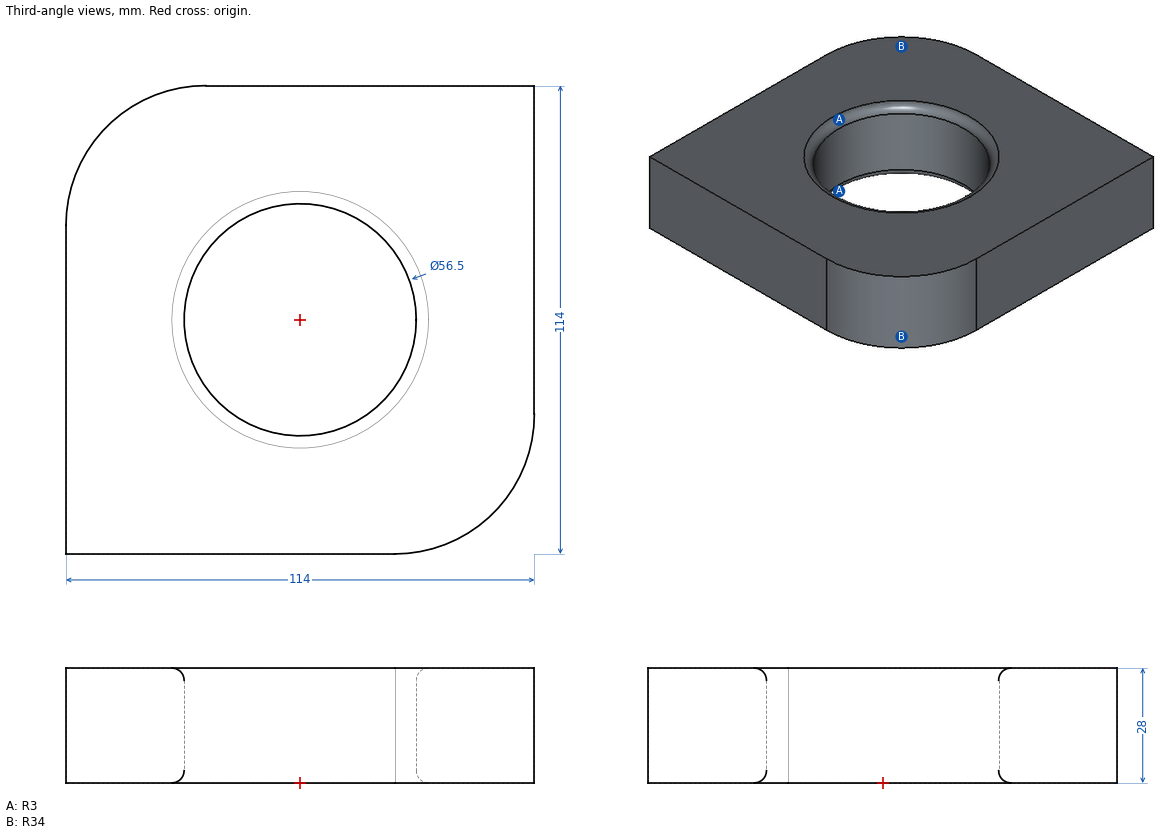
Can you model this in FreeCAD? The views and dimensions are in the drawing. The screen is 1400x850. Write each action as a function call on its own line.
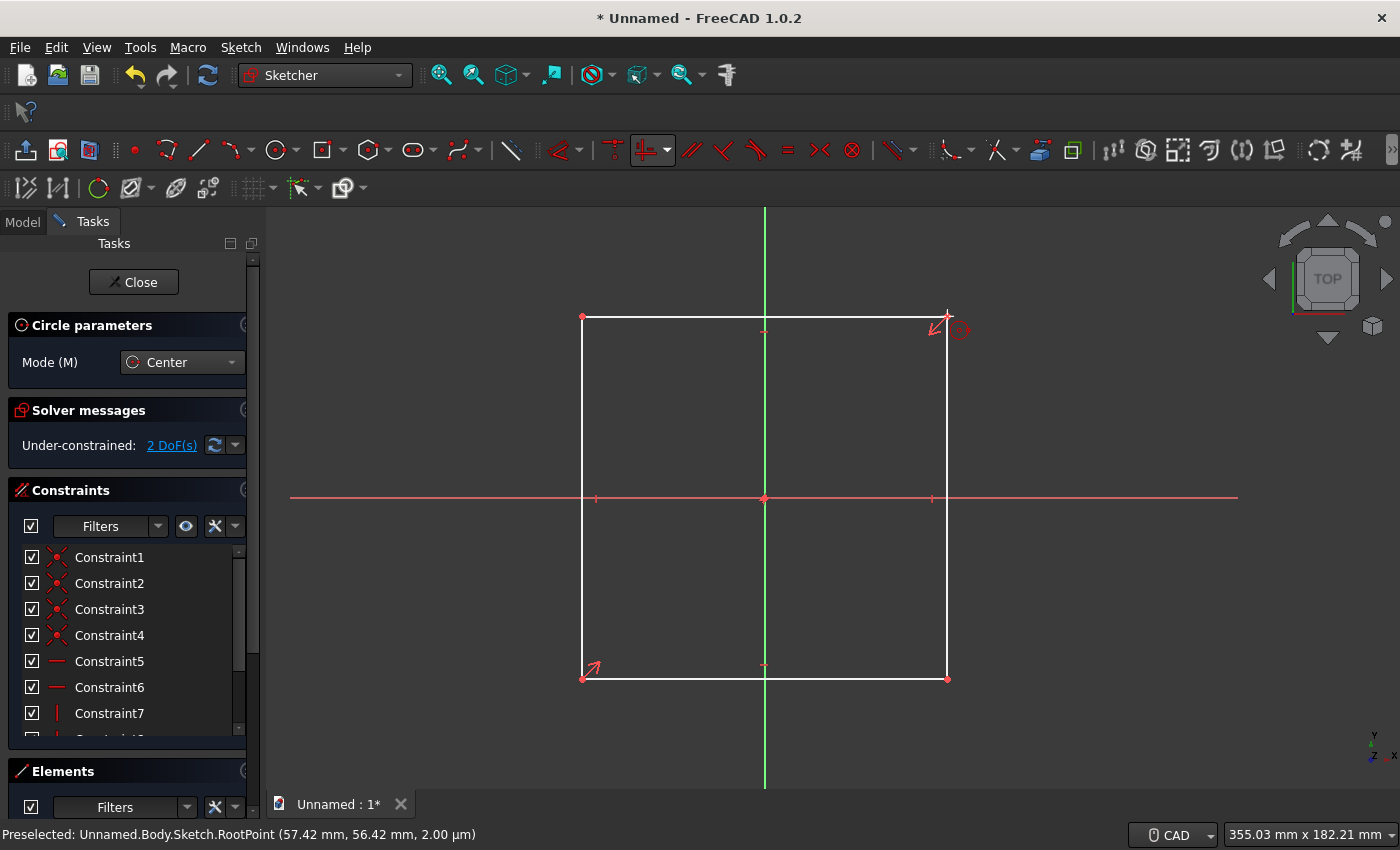
click(765, 498)
click(828, 434)
key(Escape)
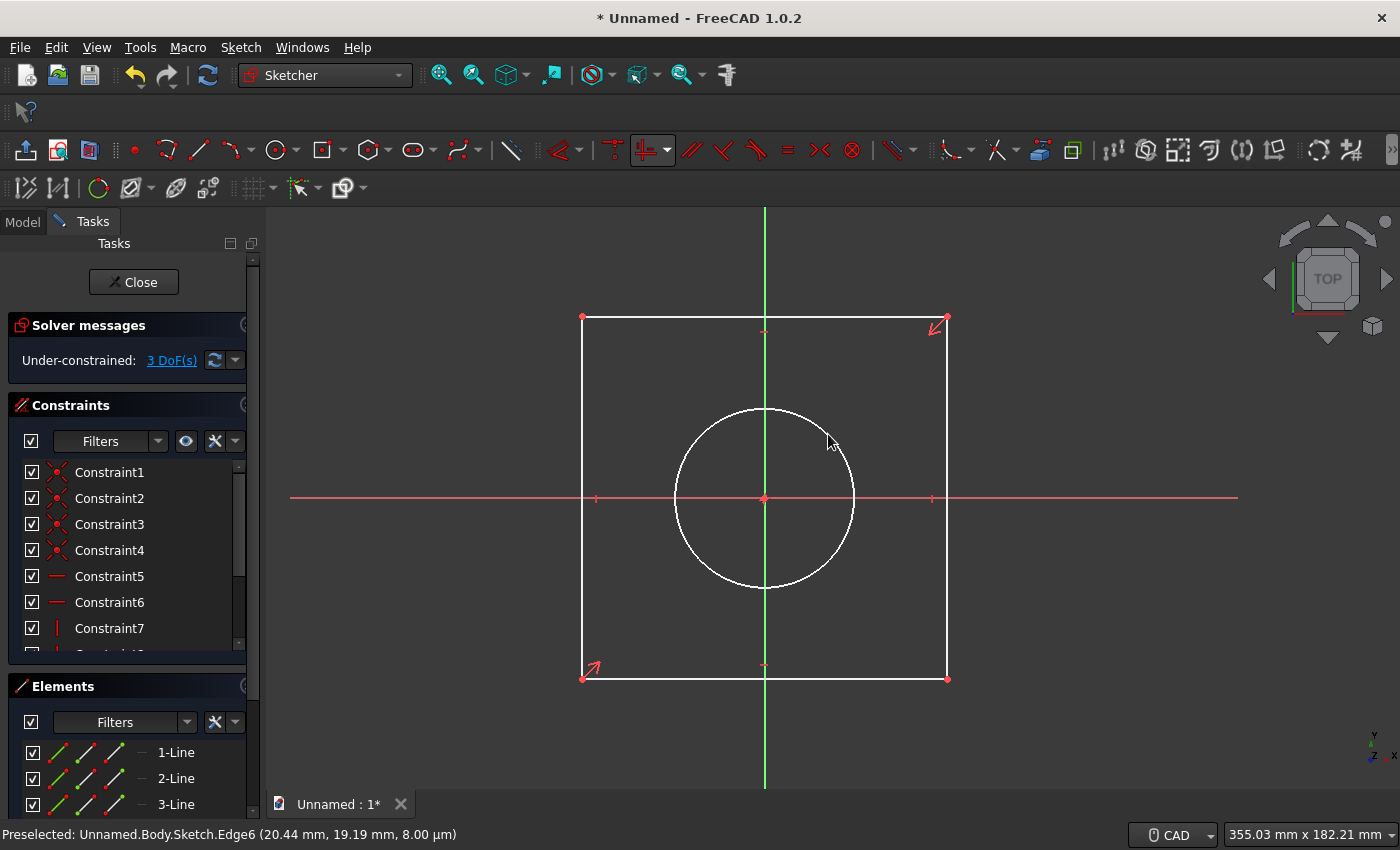
click(828, 435)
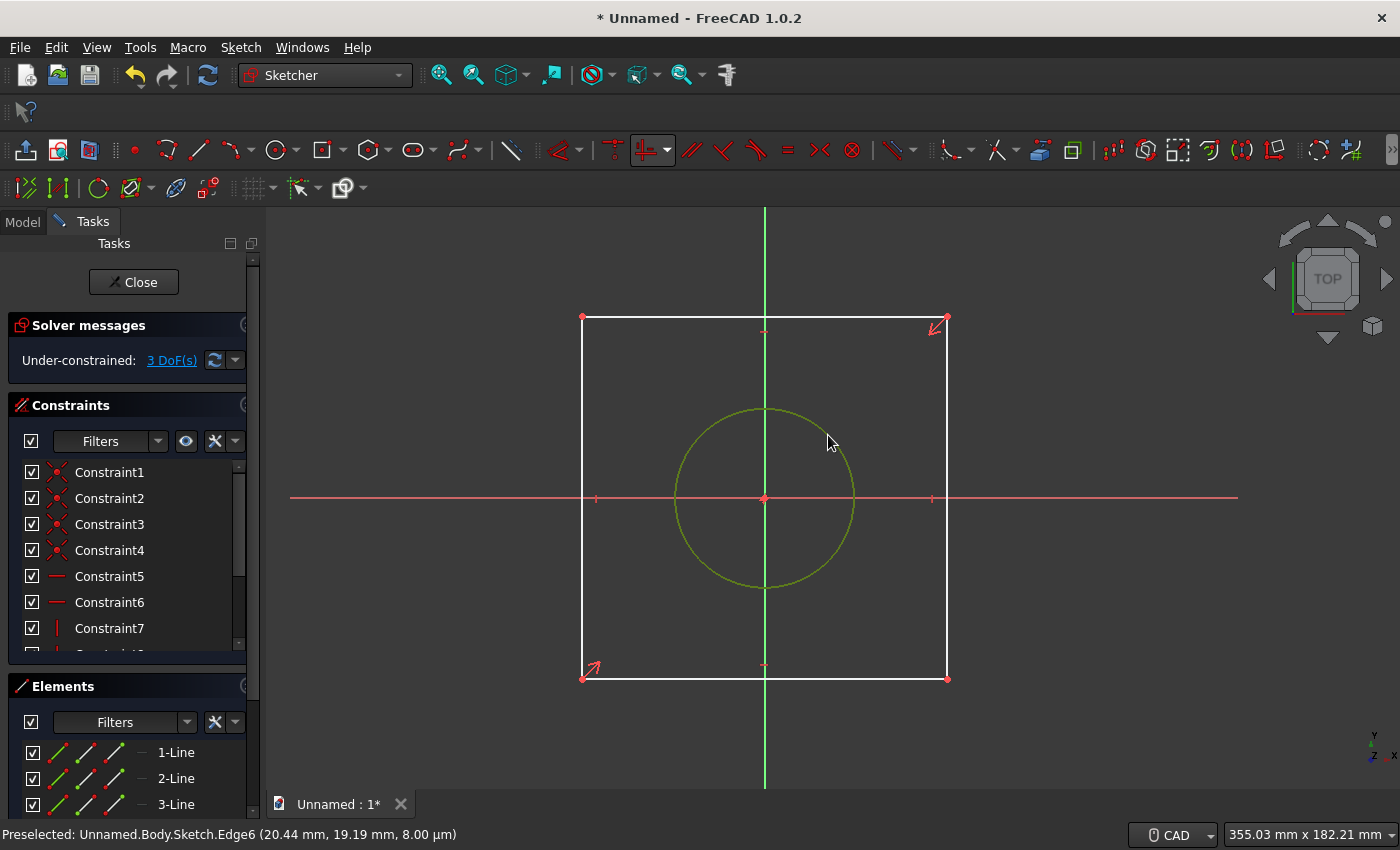
key(k)
key(o)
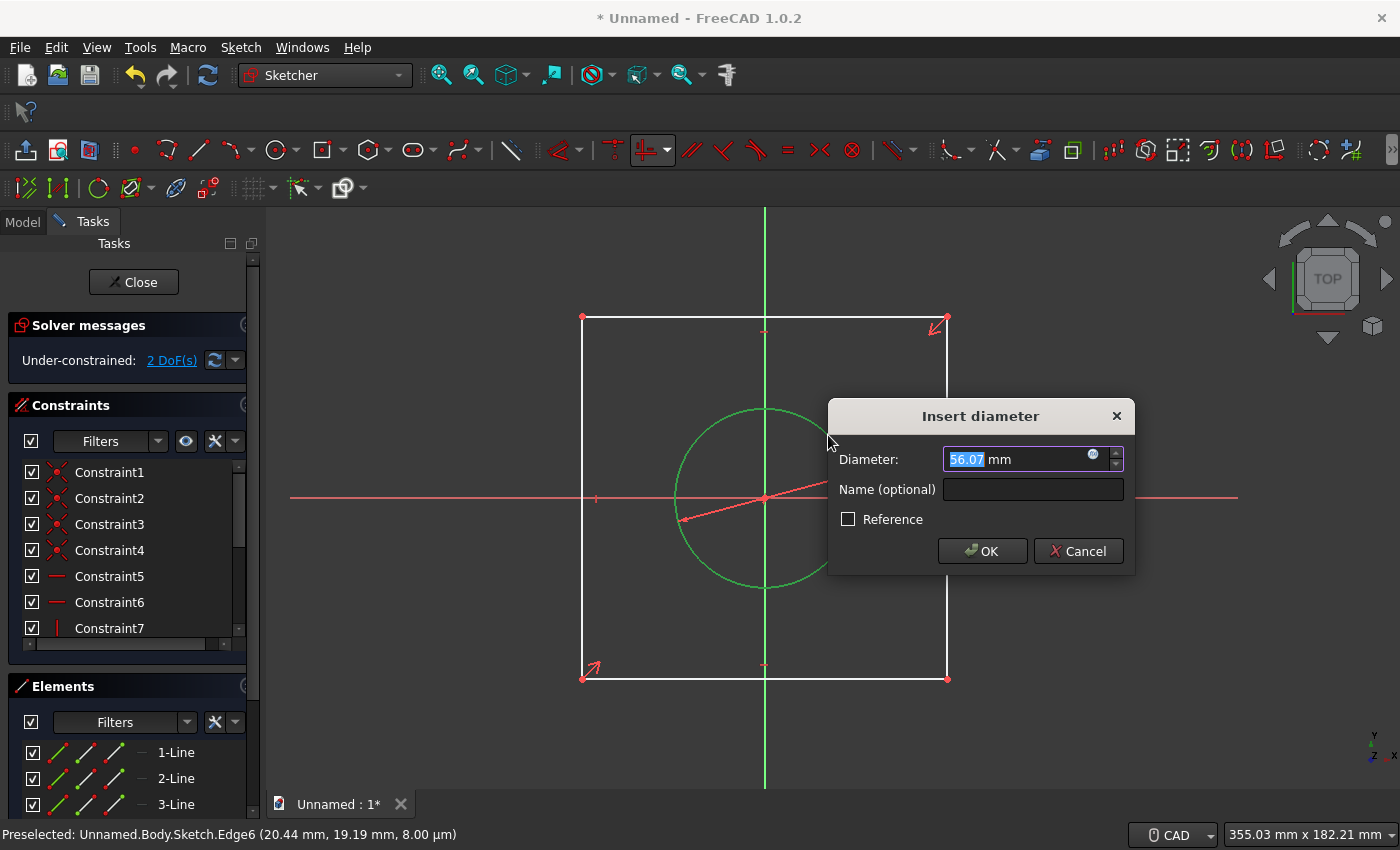
text(56.5)
key(Return)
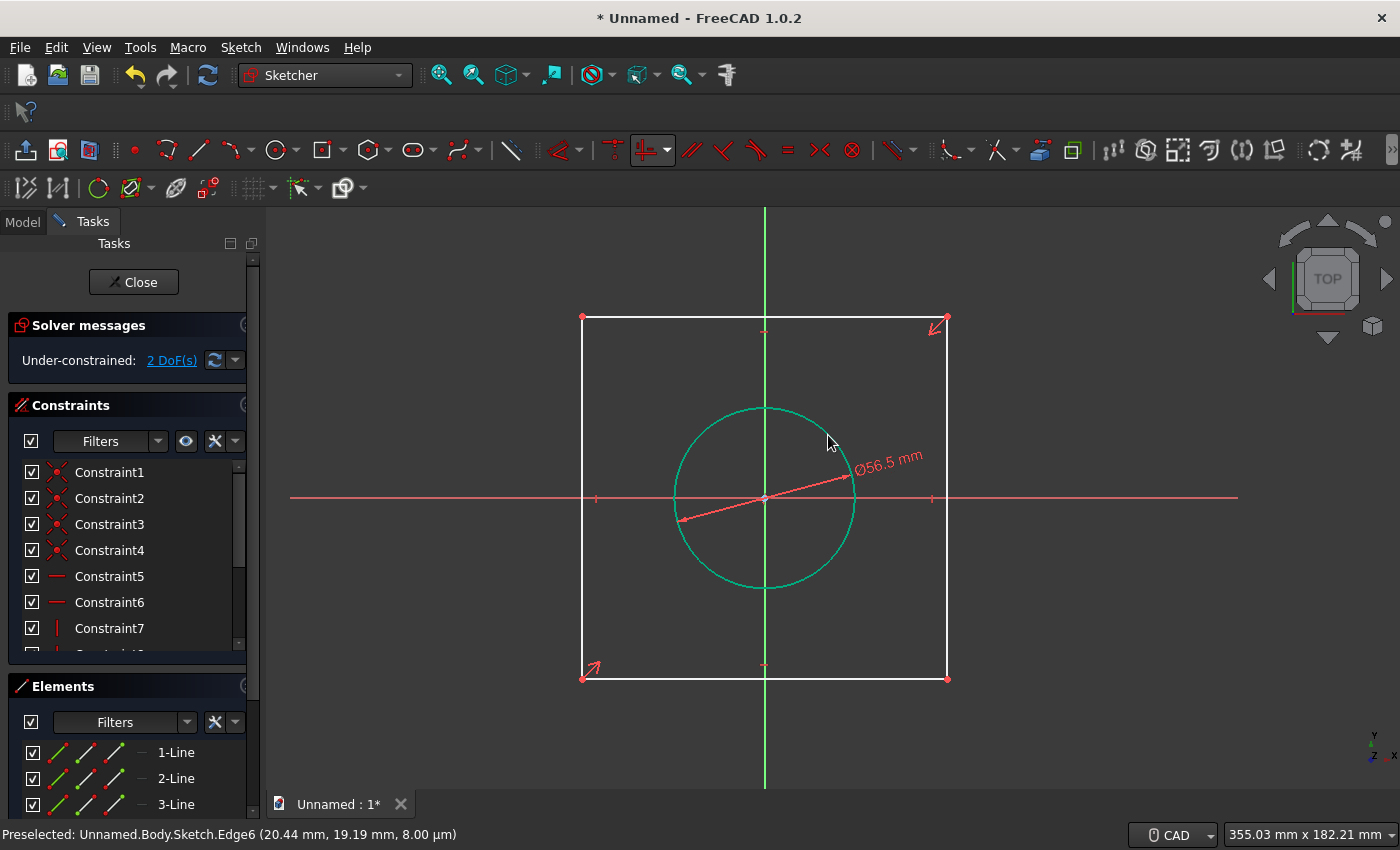
click(692, 679)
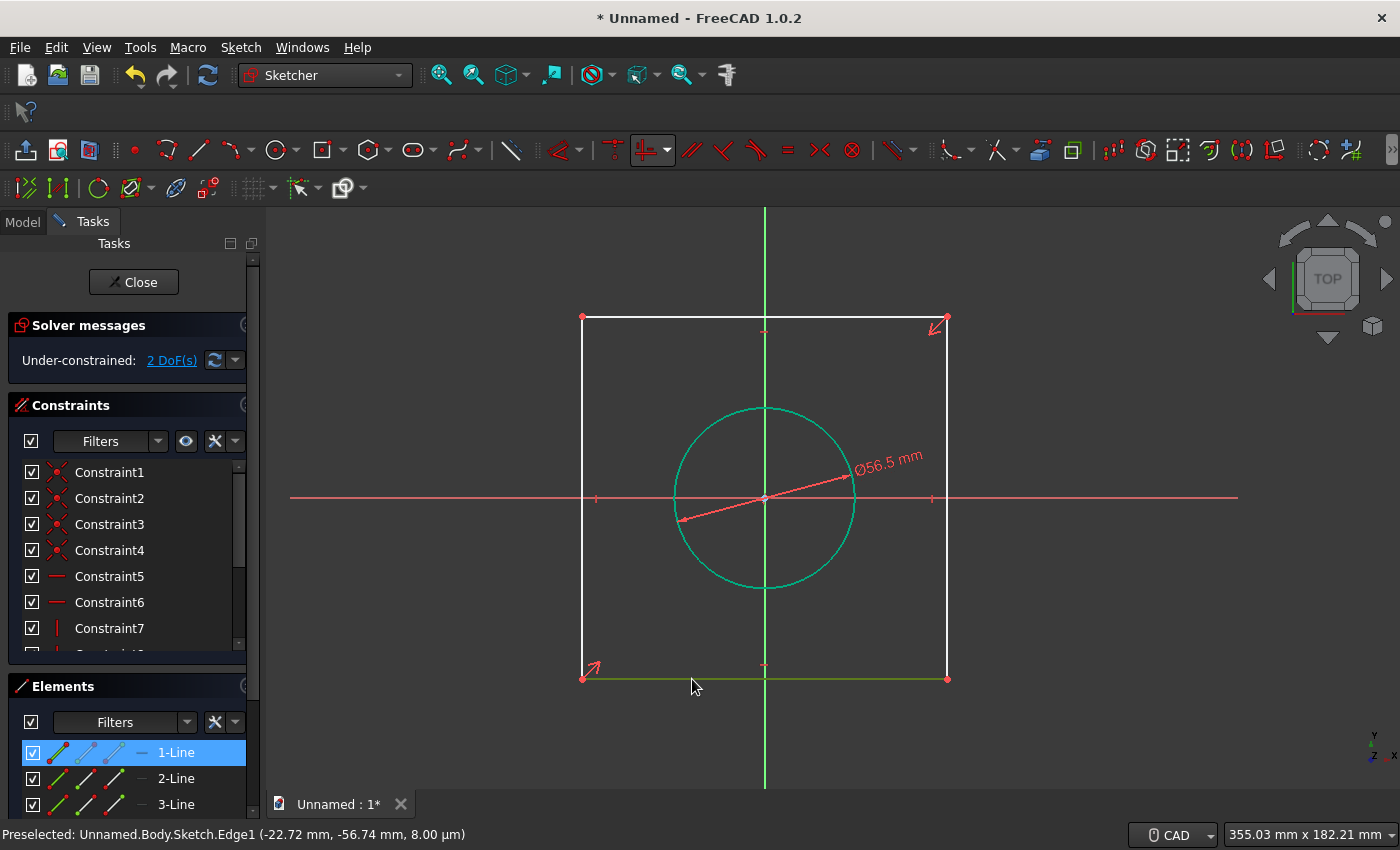
key(l)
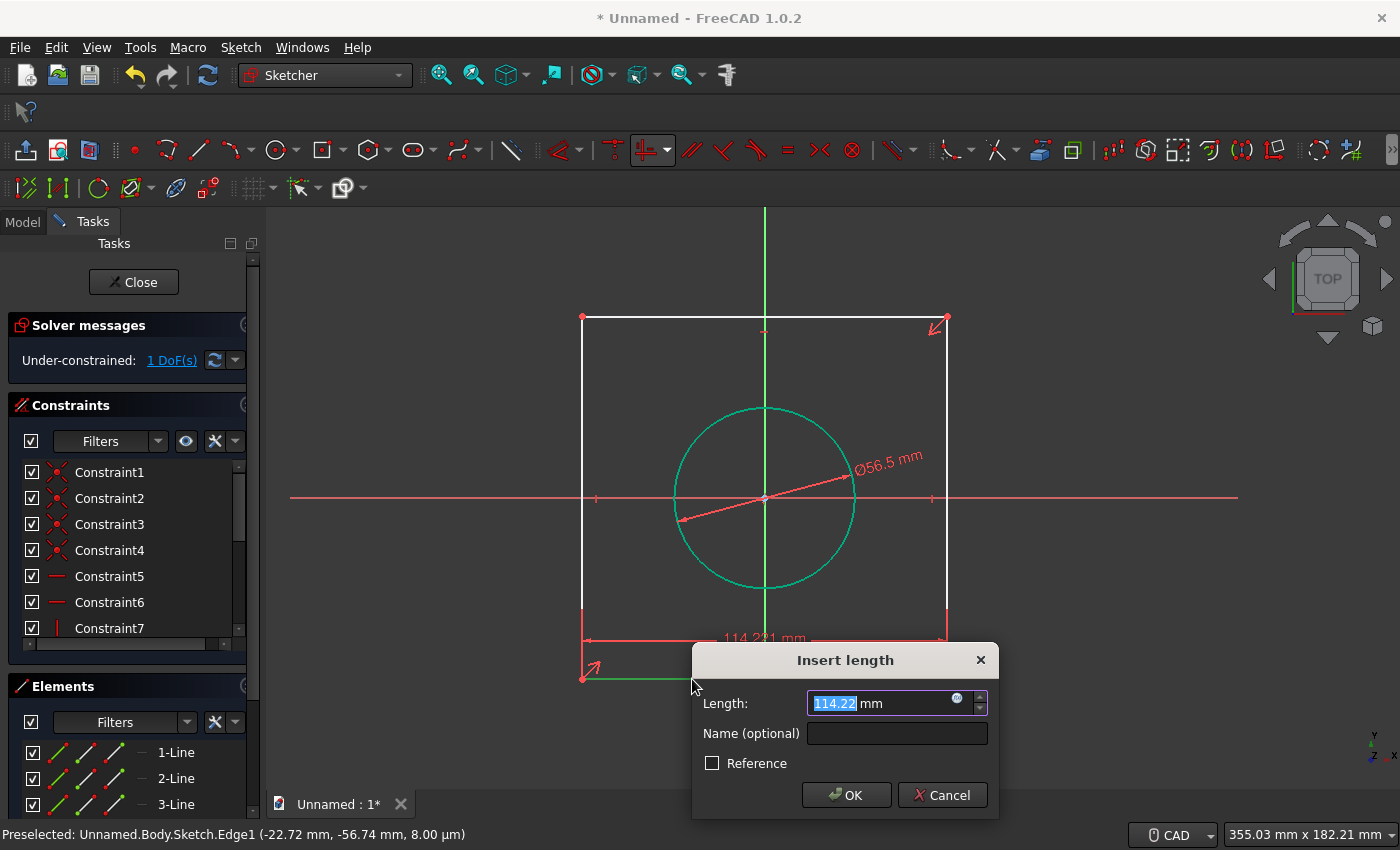
text(114)
key(Return)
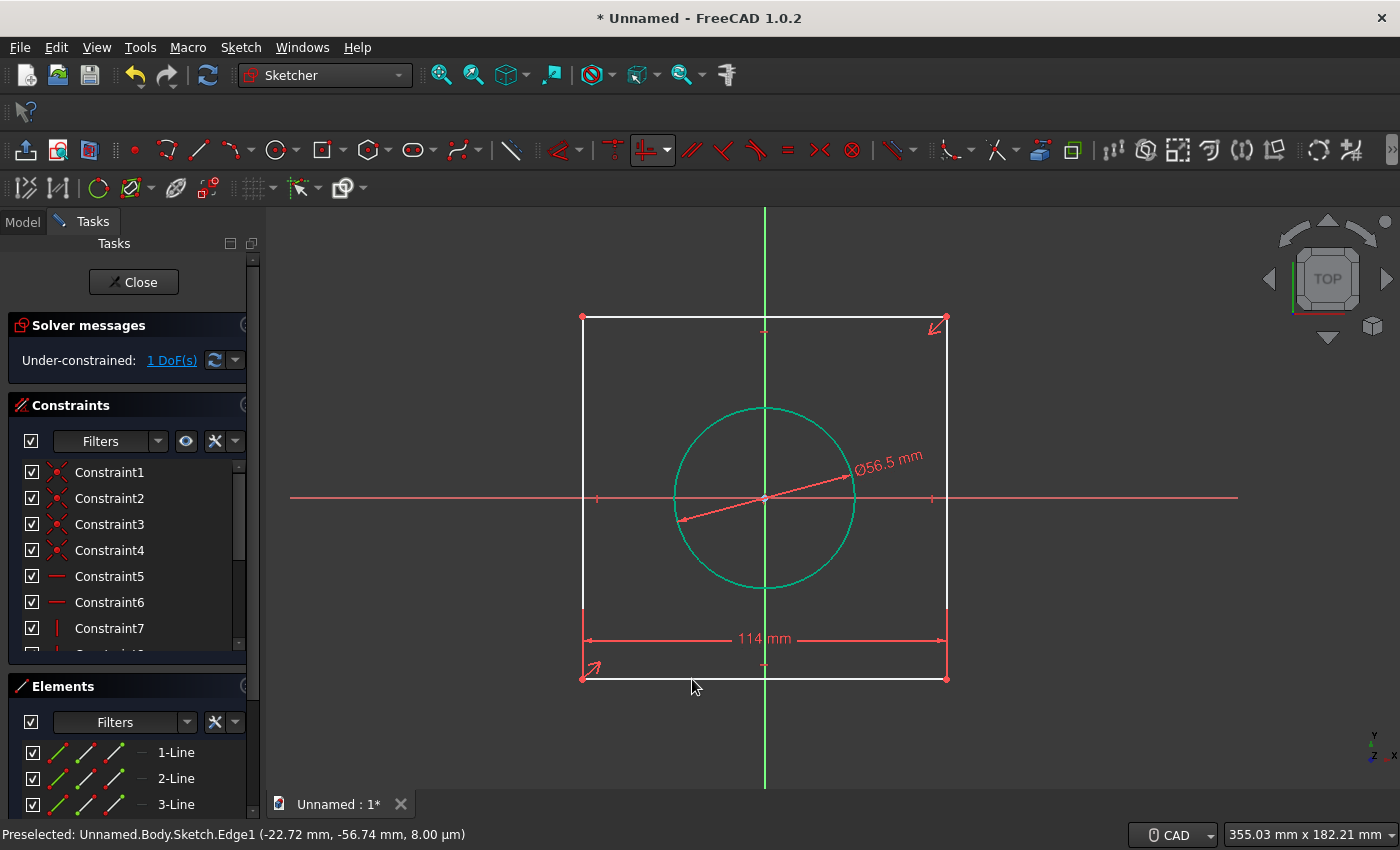
click(947, 571)